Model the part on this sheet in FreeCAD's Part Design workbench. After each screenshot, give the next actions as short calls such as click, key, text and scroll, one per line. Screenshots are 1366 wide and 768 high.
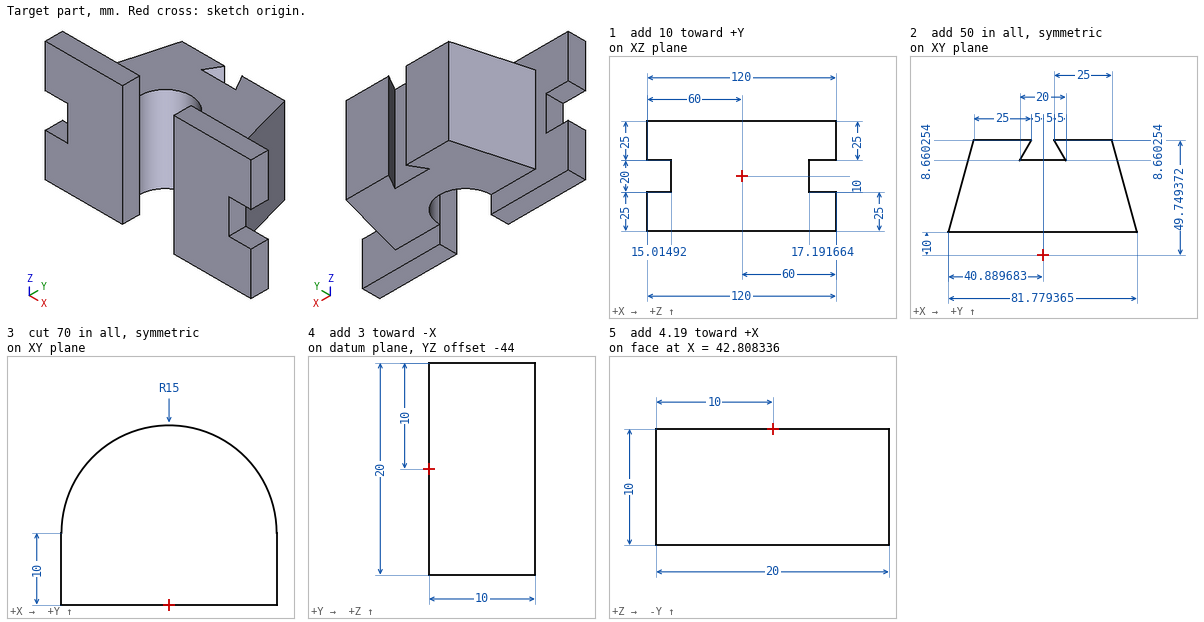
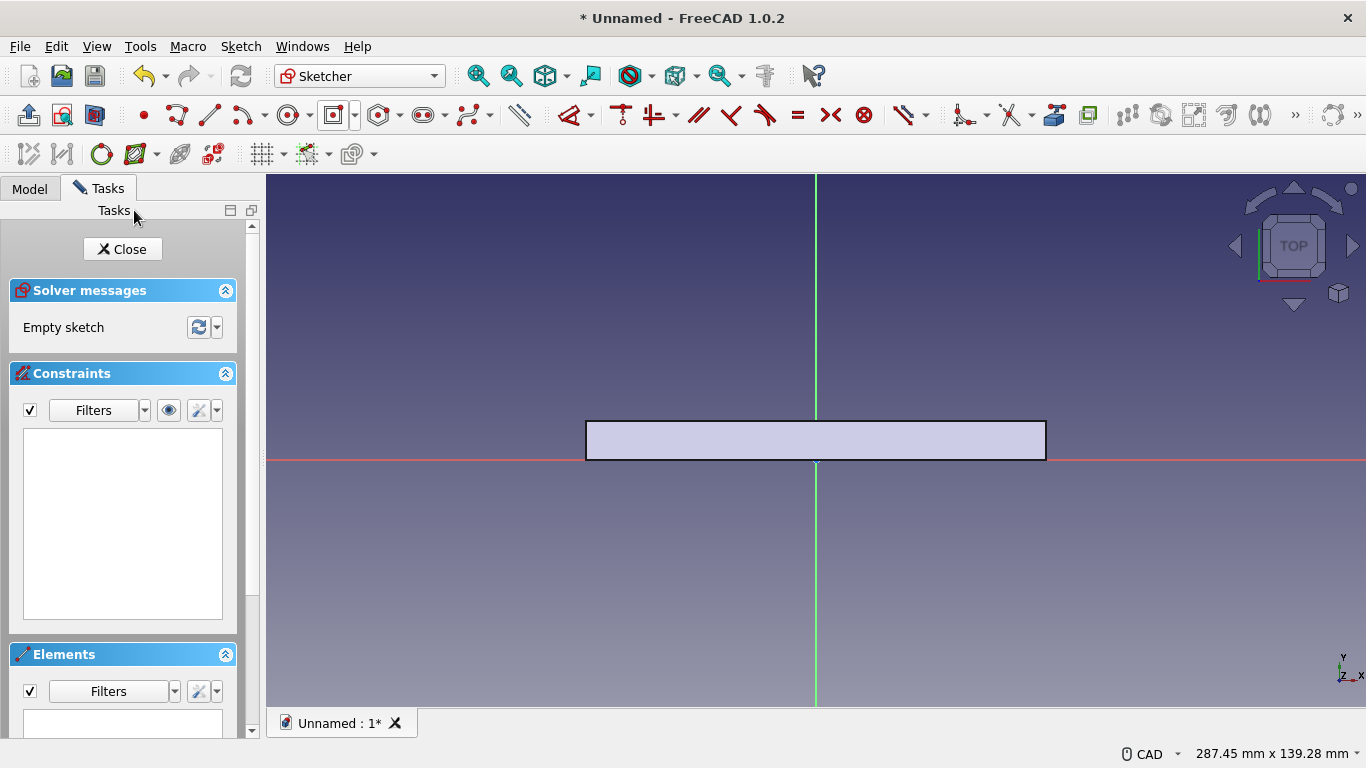
key(q)
key(s)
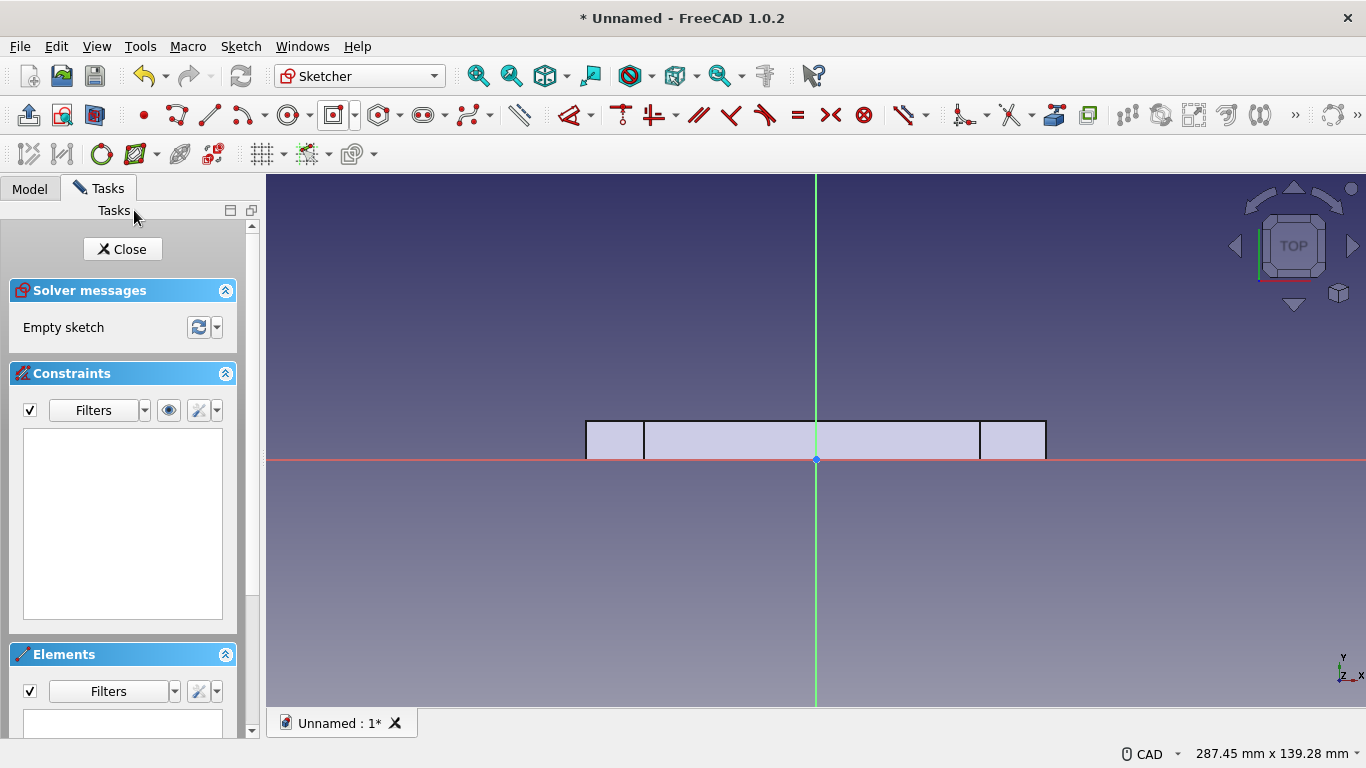
scroll(899, 272, up, 3)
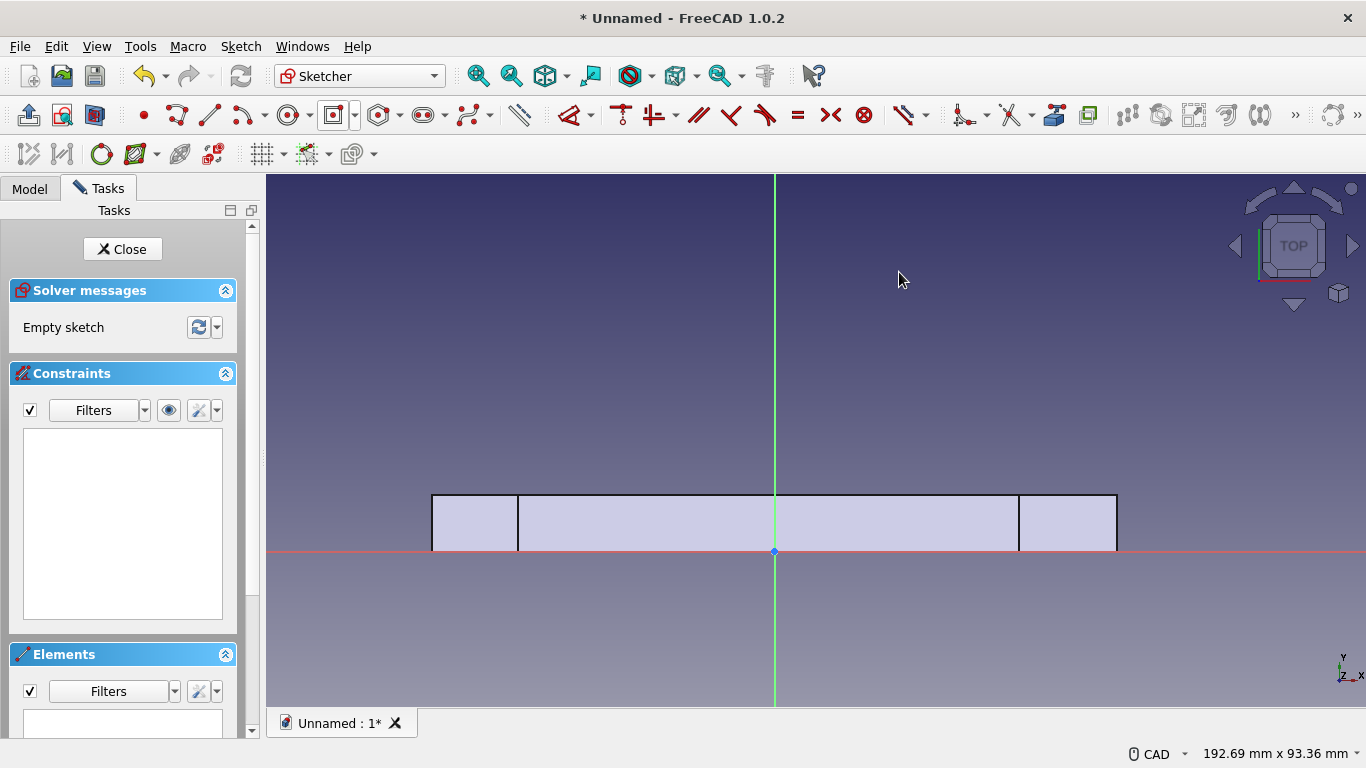
key(g)
key(m)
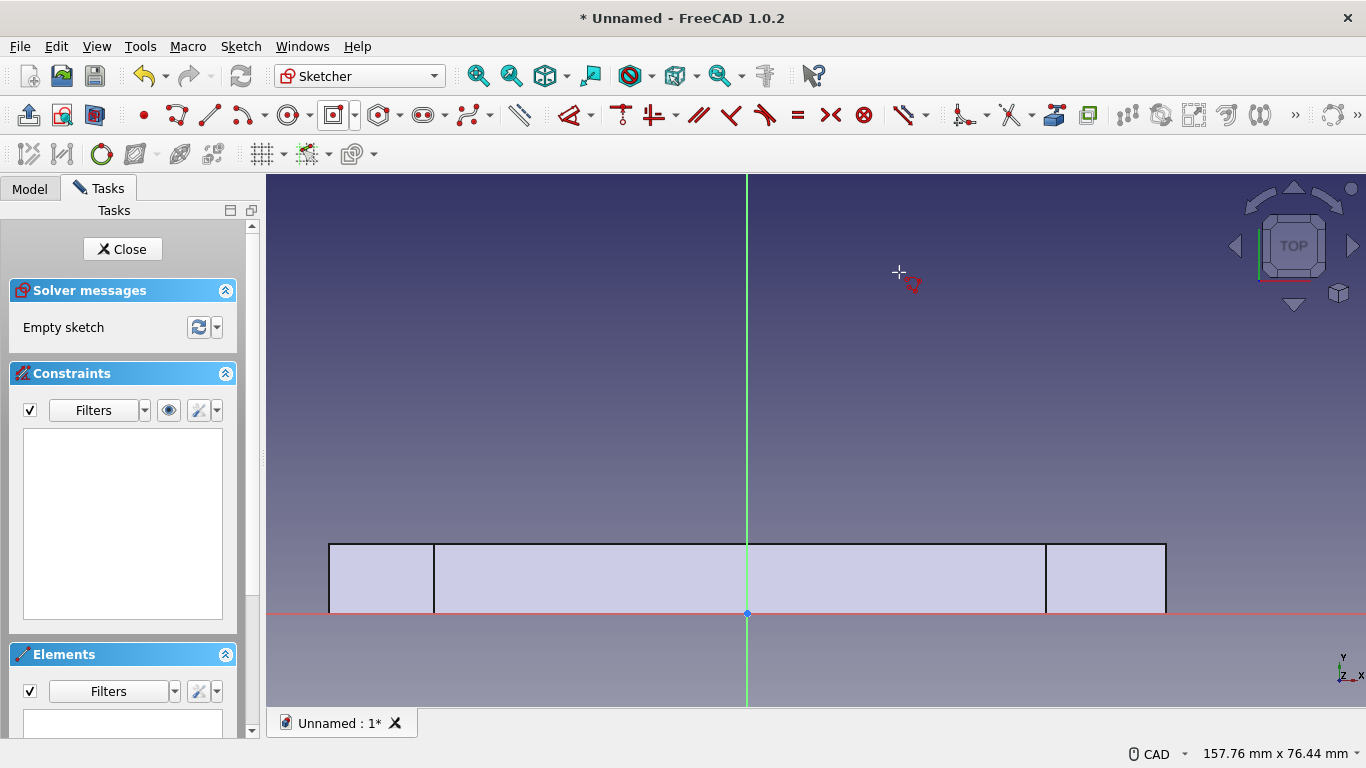
click(462, 544)
click(1032, 544)
click(956, 267)
click(782, 267)
click(817, 327)
click(678, 327)
click(712, 267)
click(538, 267)
click(462, 545)
key(Escape)
key(Escape)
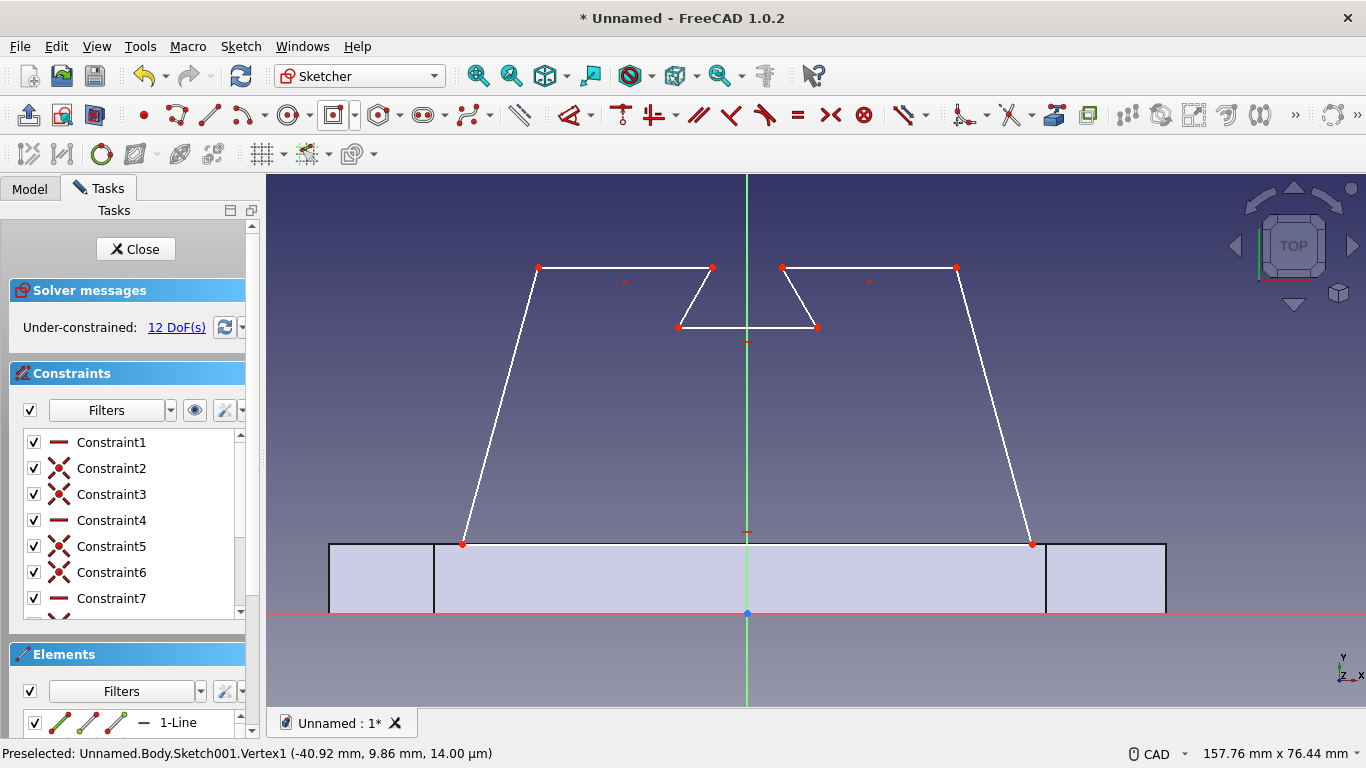
key(d)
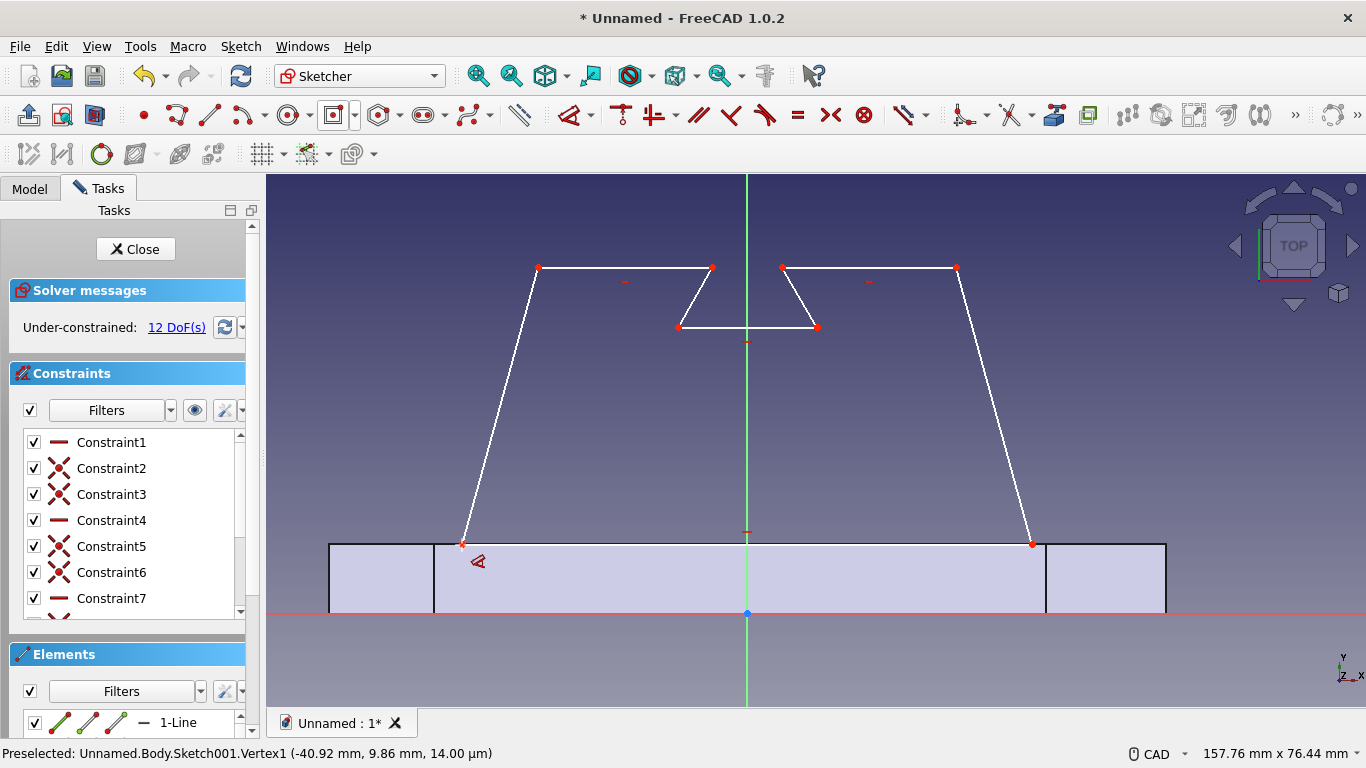
click(904, 268)
click(869, 234)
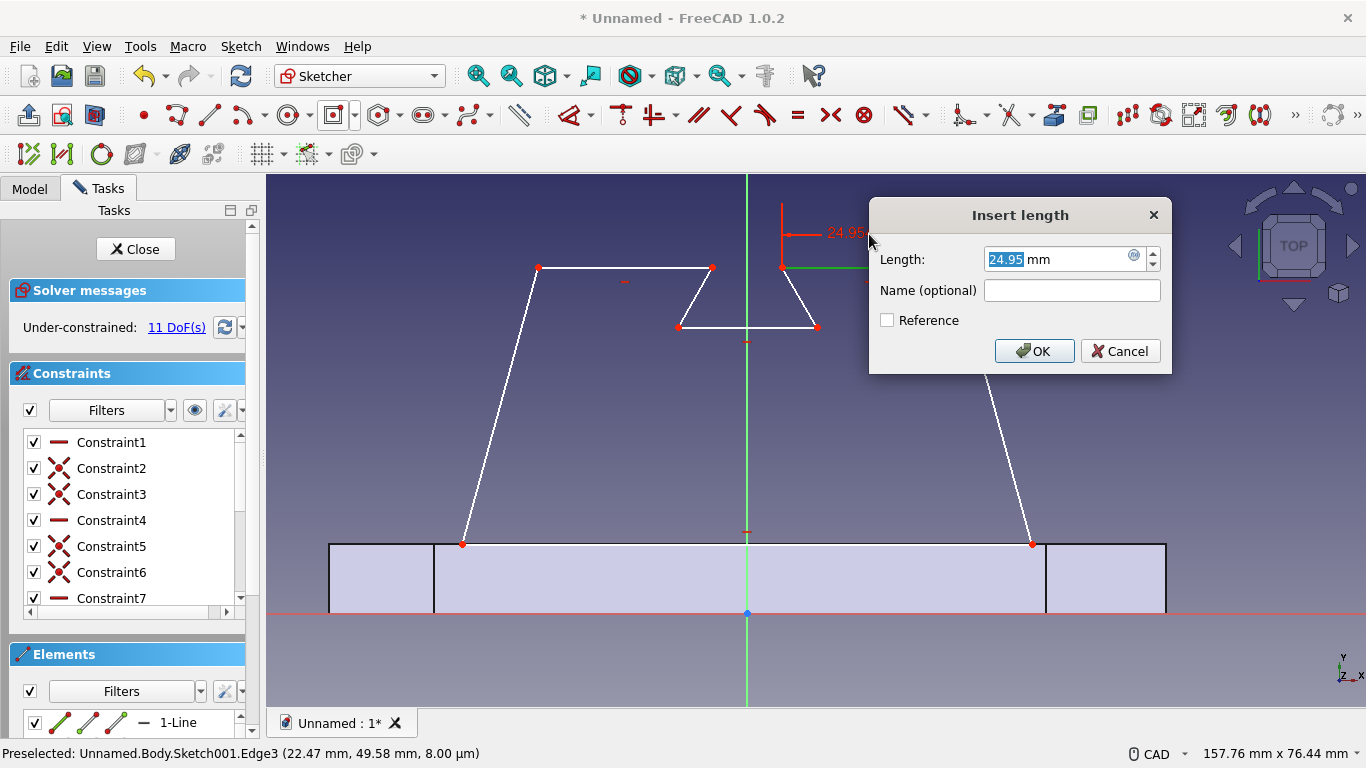
text(25)
key(Return)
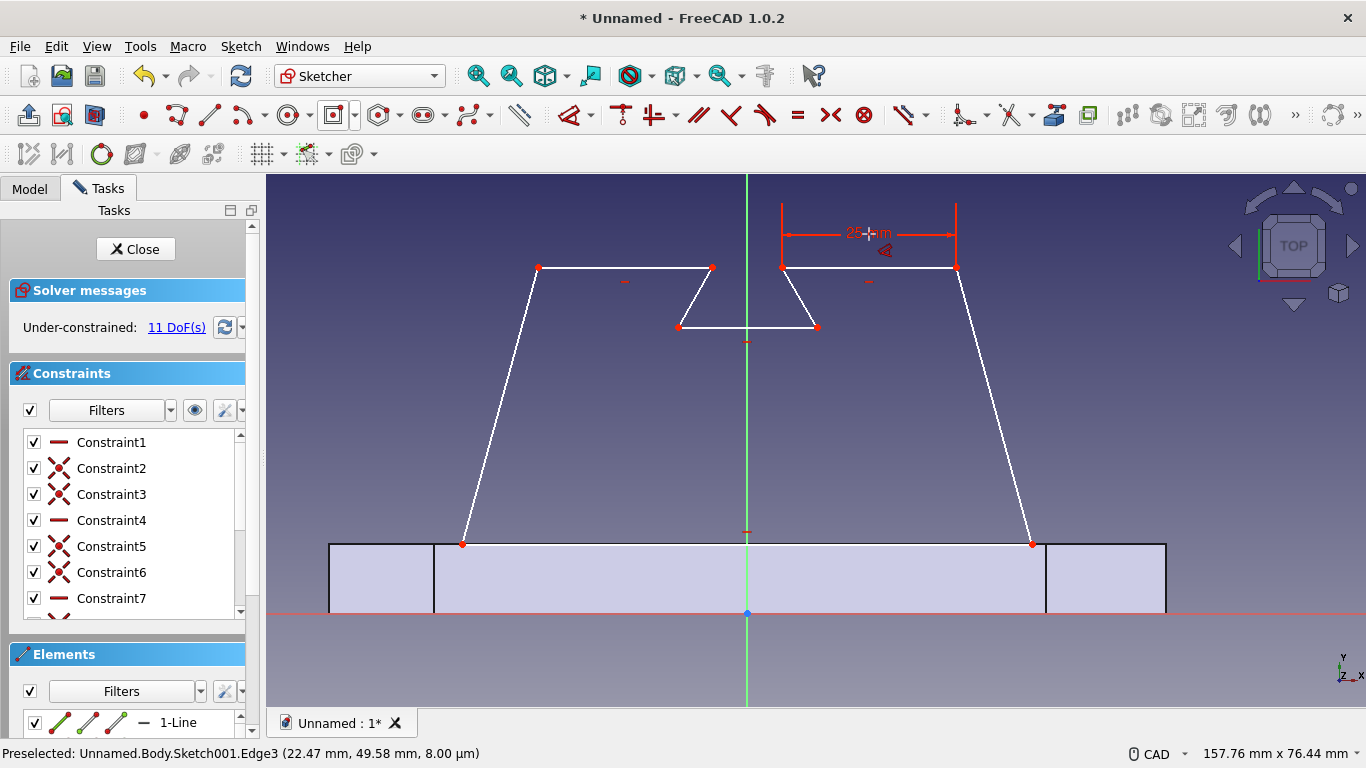
click(775, 328)
click(716, 294)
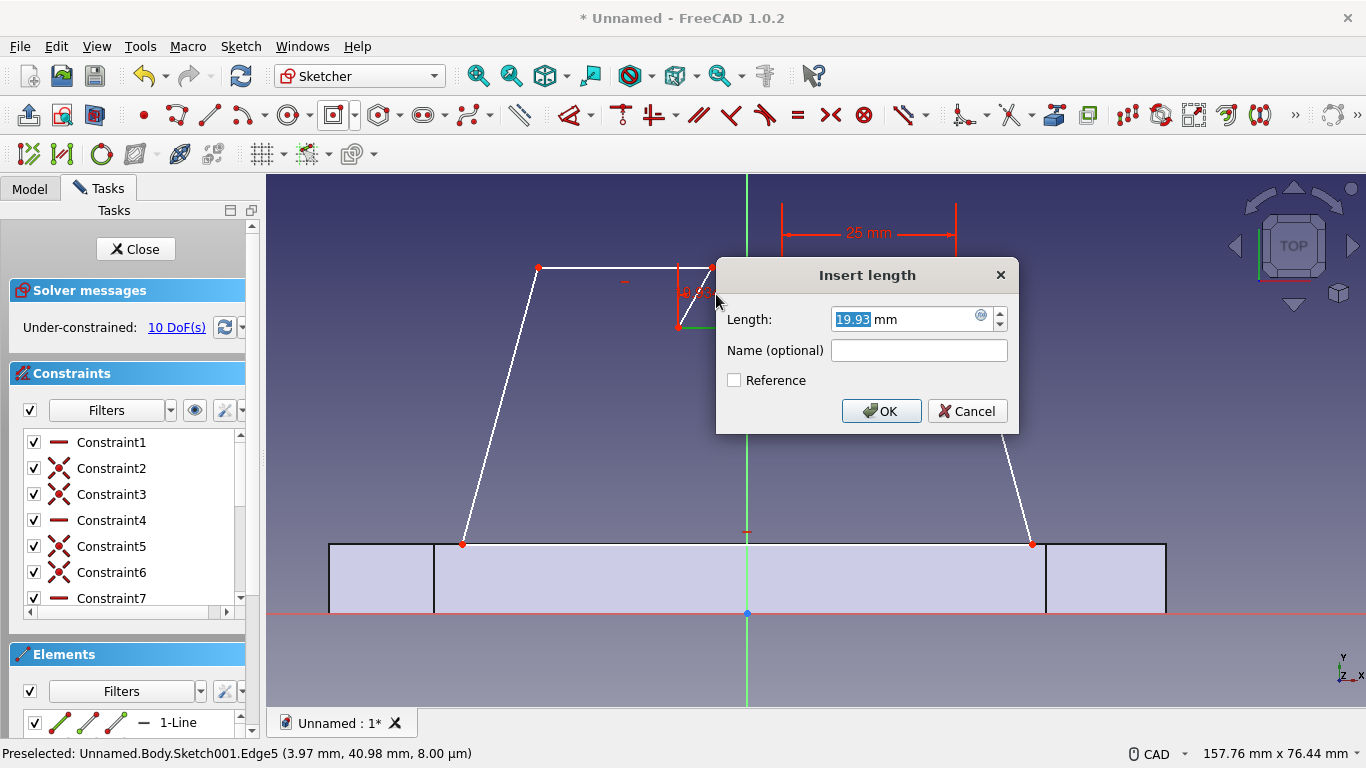
text(20)
key(Return)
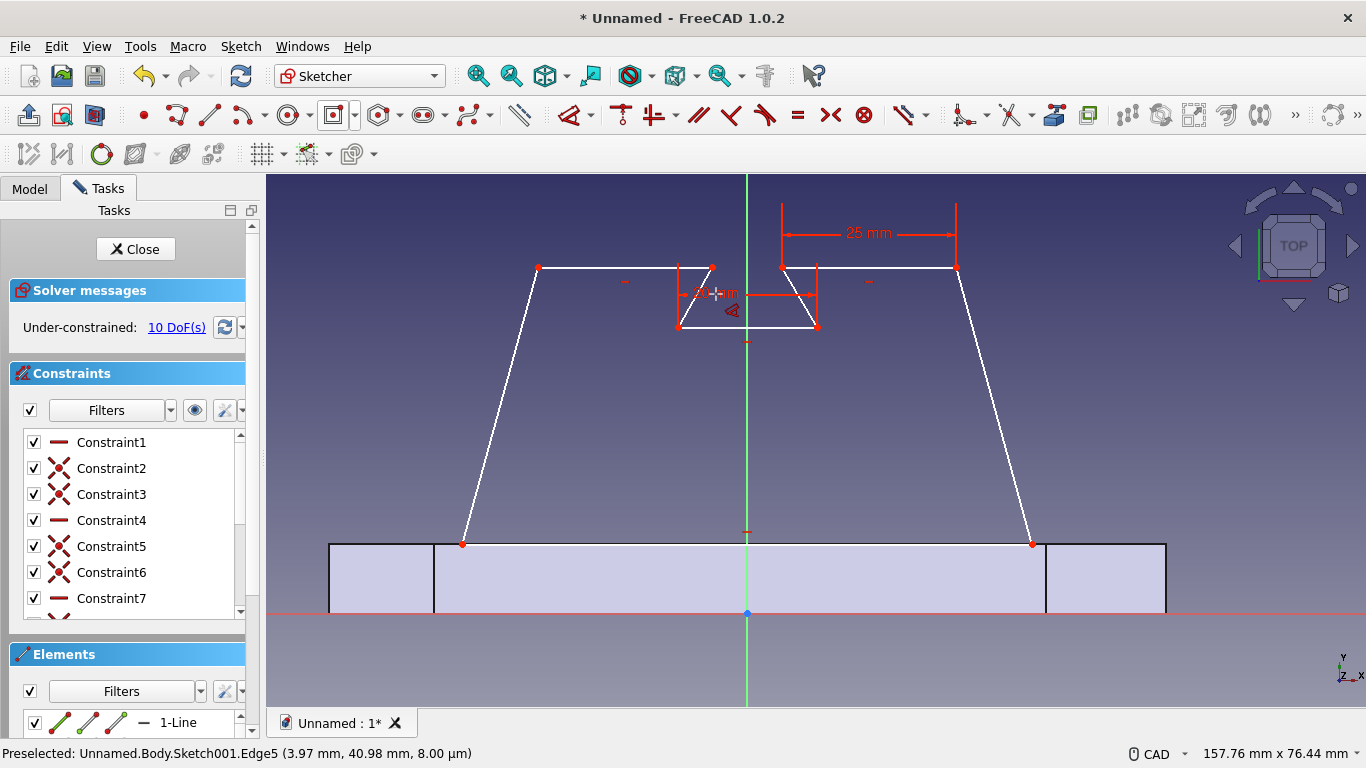
click(660, 268)
click(625, 234)